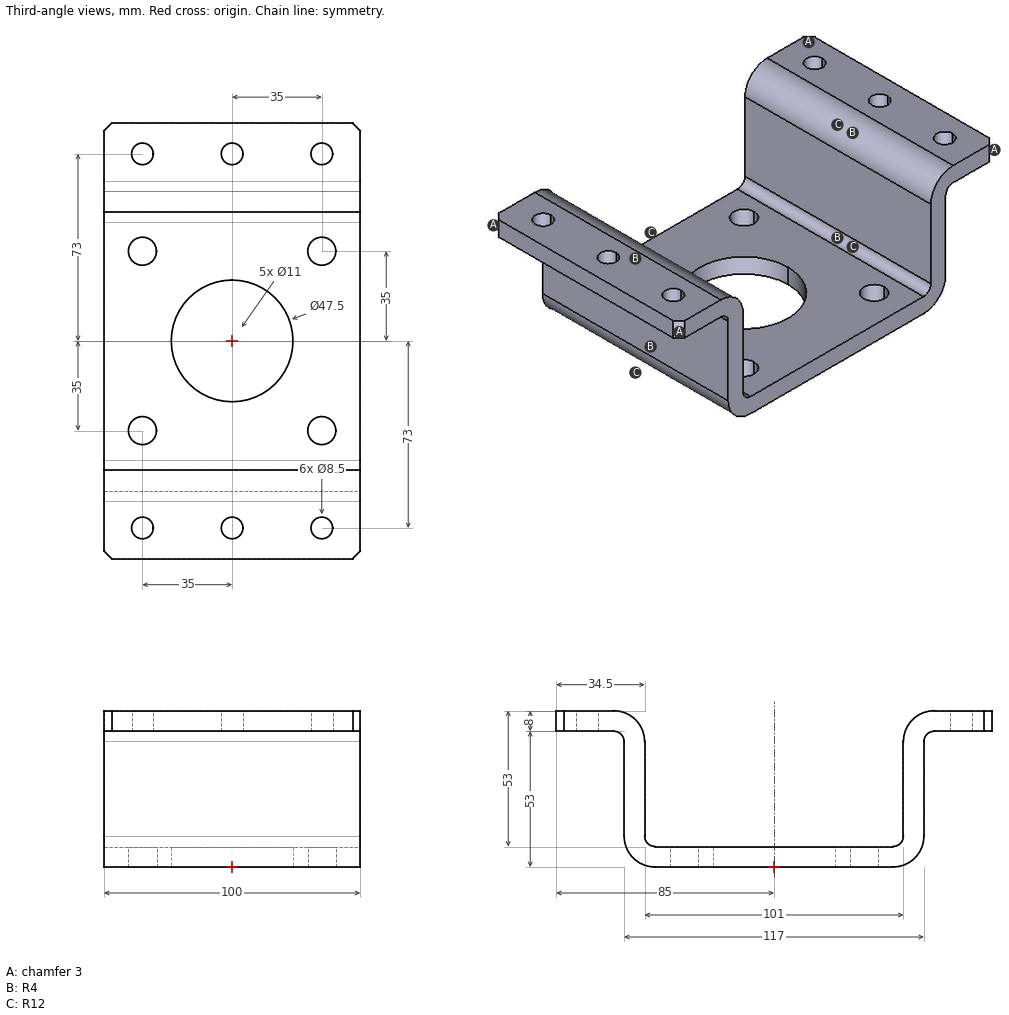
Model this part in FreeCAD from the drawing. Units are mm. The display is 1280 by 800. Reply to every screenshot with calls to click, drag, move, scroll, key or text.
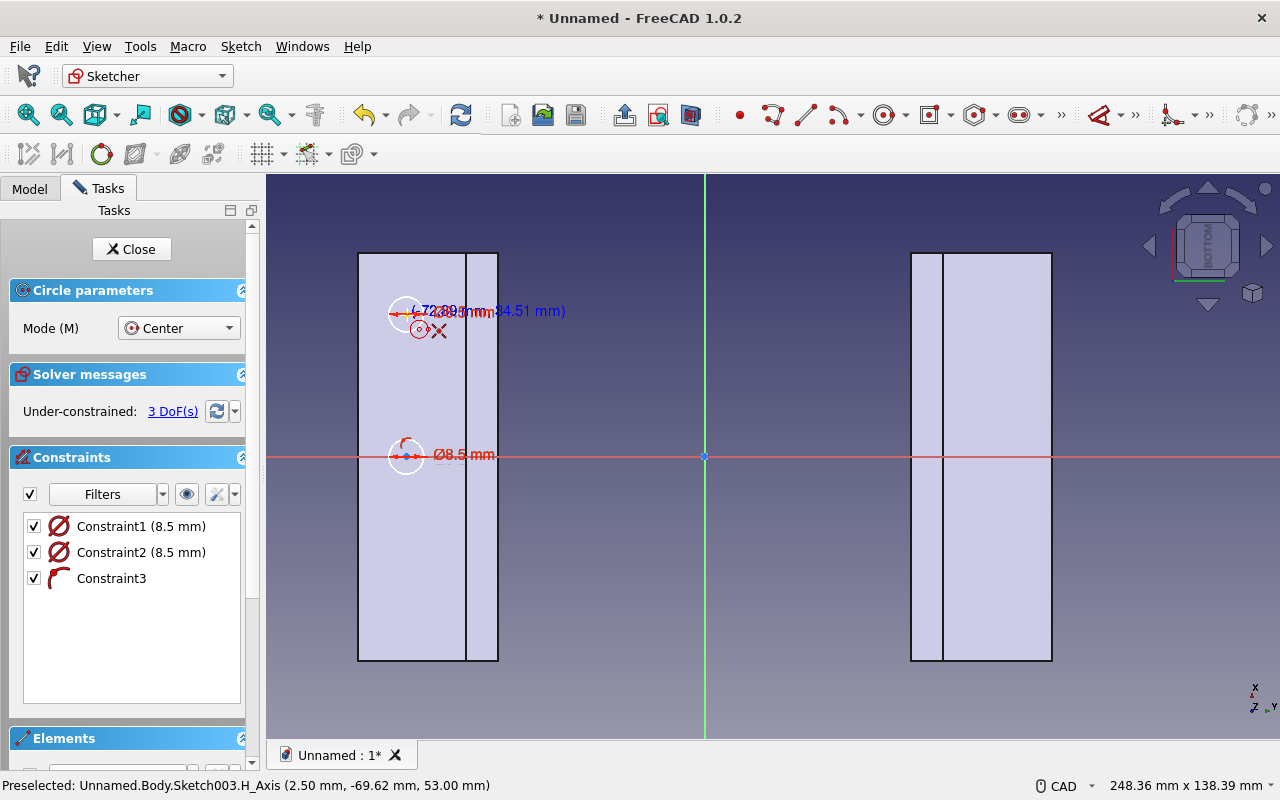
scroll(407, 600, up, 2)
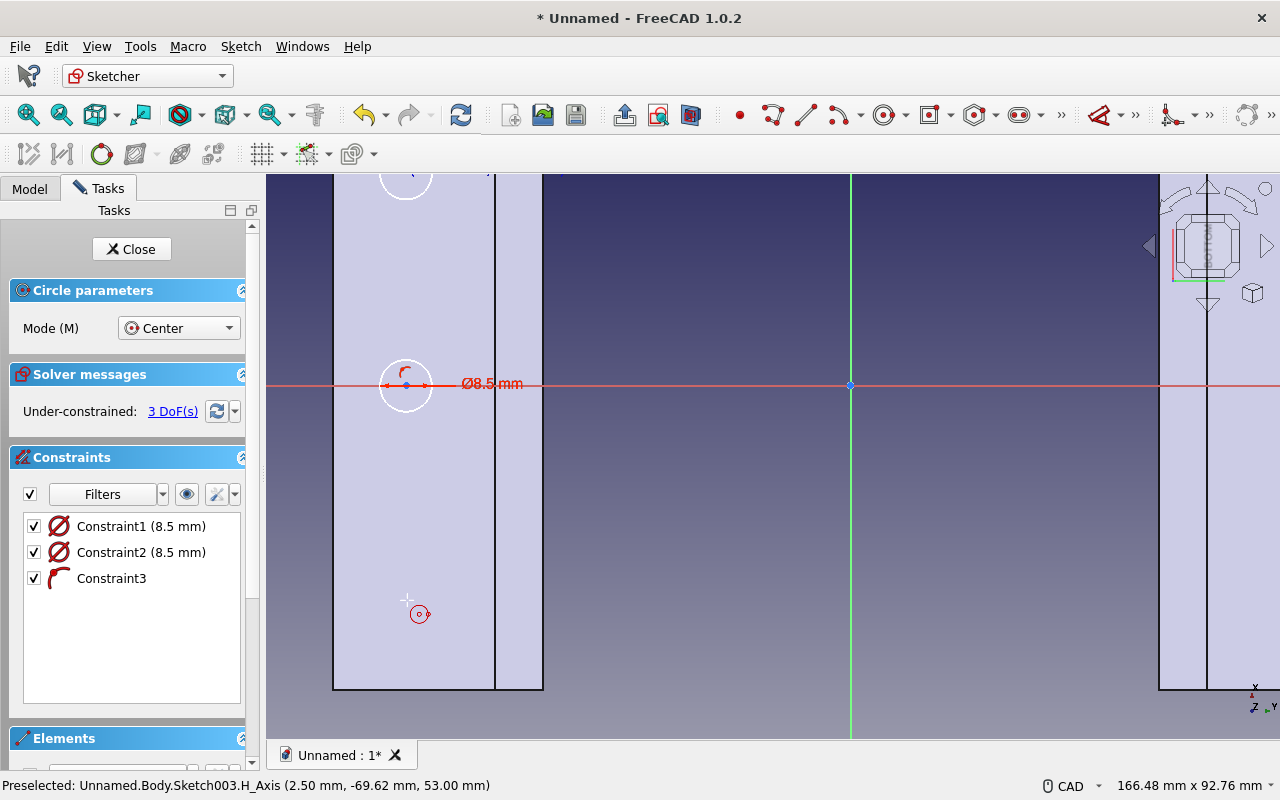
click(406, 599)
move(425, 581)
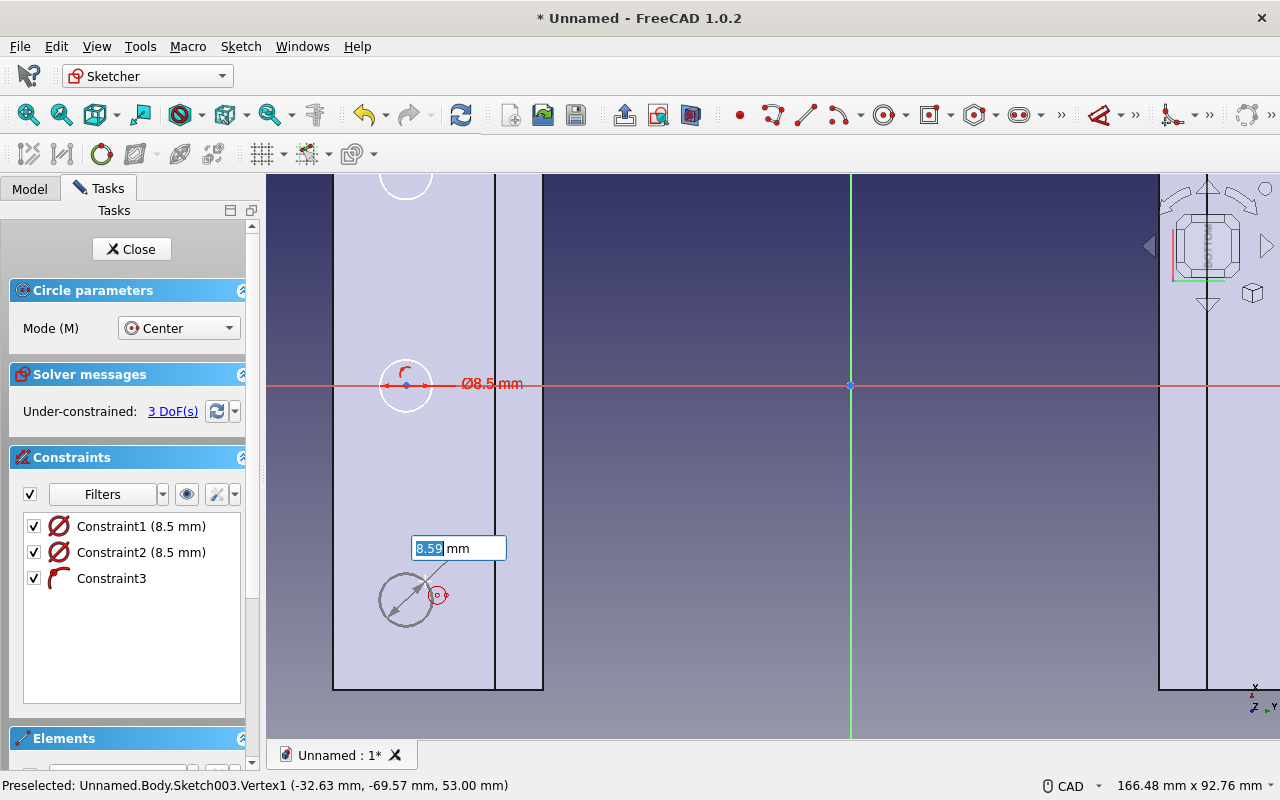
text(8.5)
key(Return)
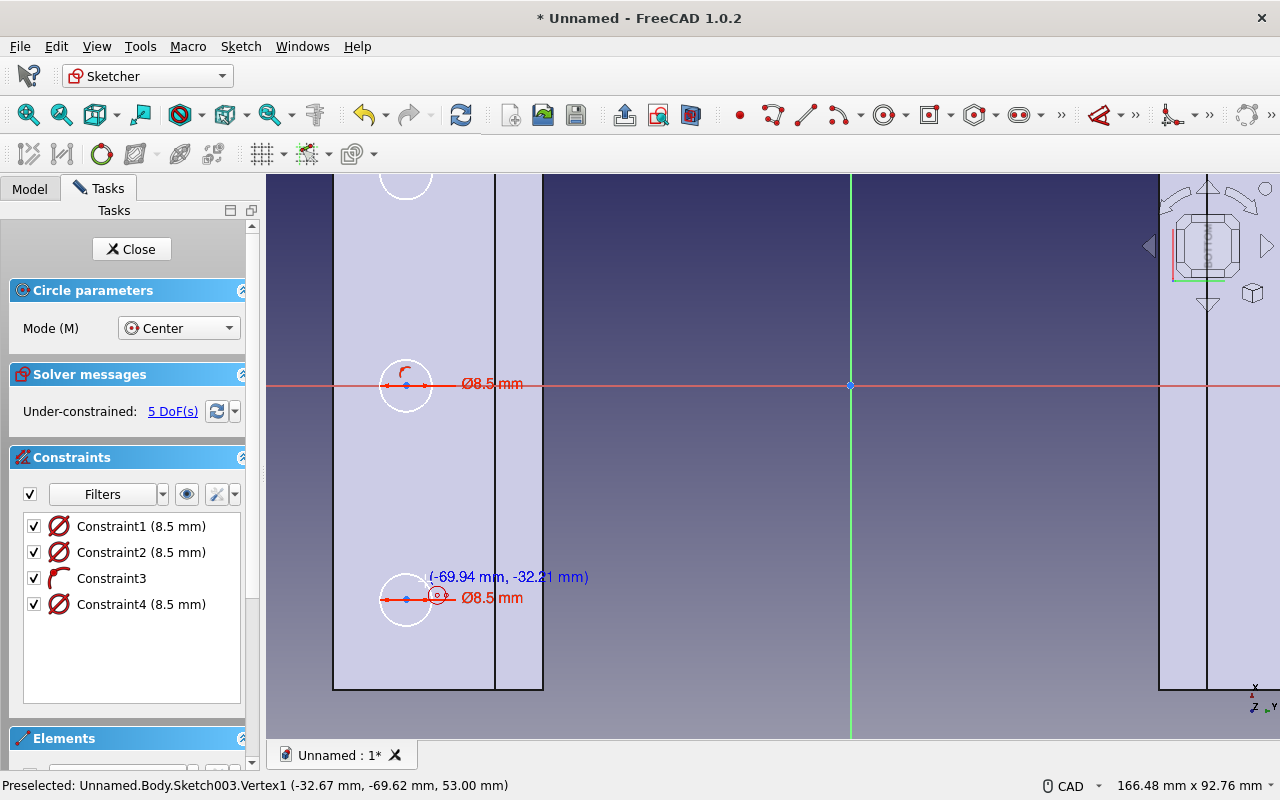
scroll(407, 600, down, 2)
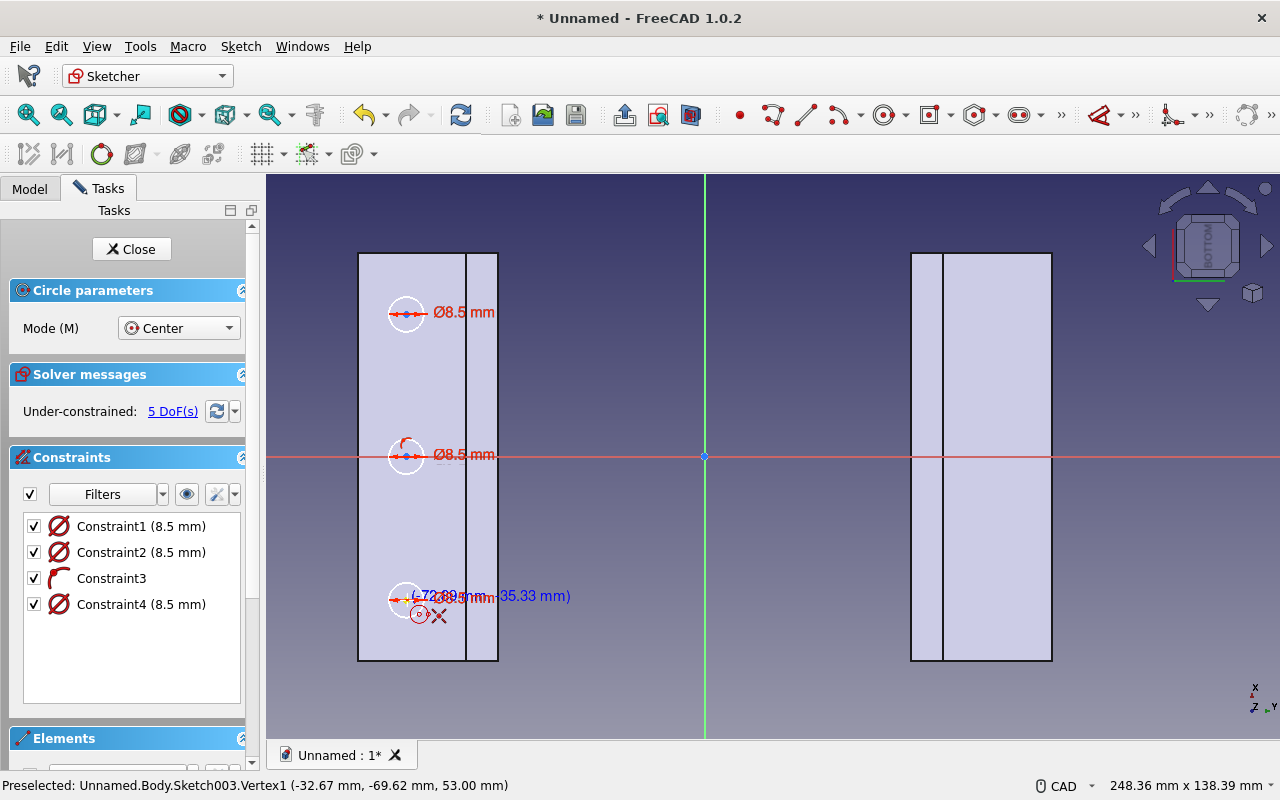
scroll(1003, 600, up, 2)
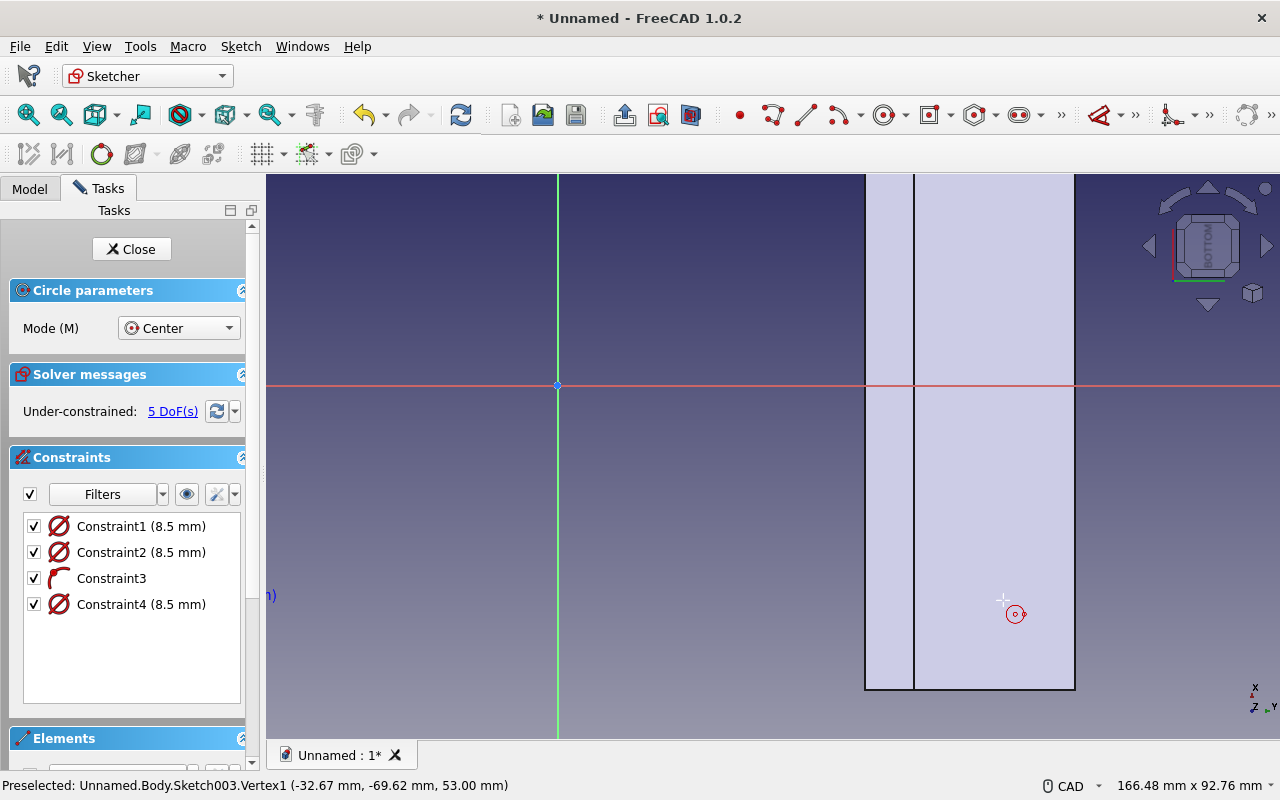
click(1002, 599)
move(1020, 581)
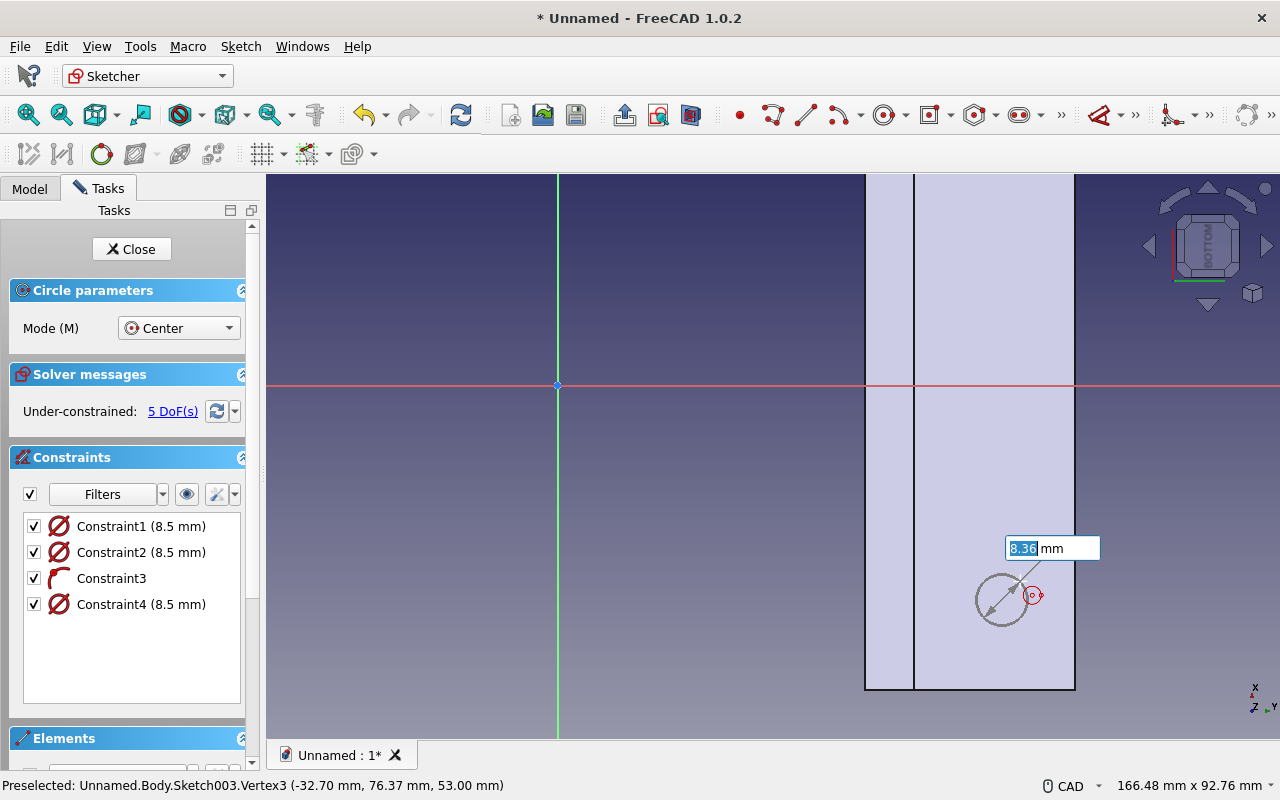
text(8.5)
key(Return)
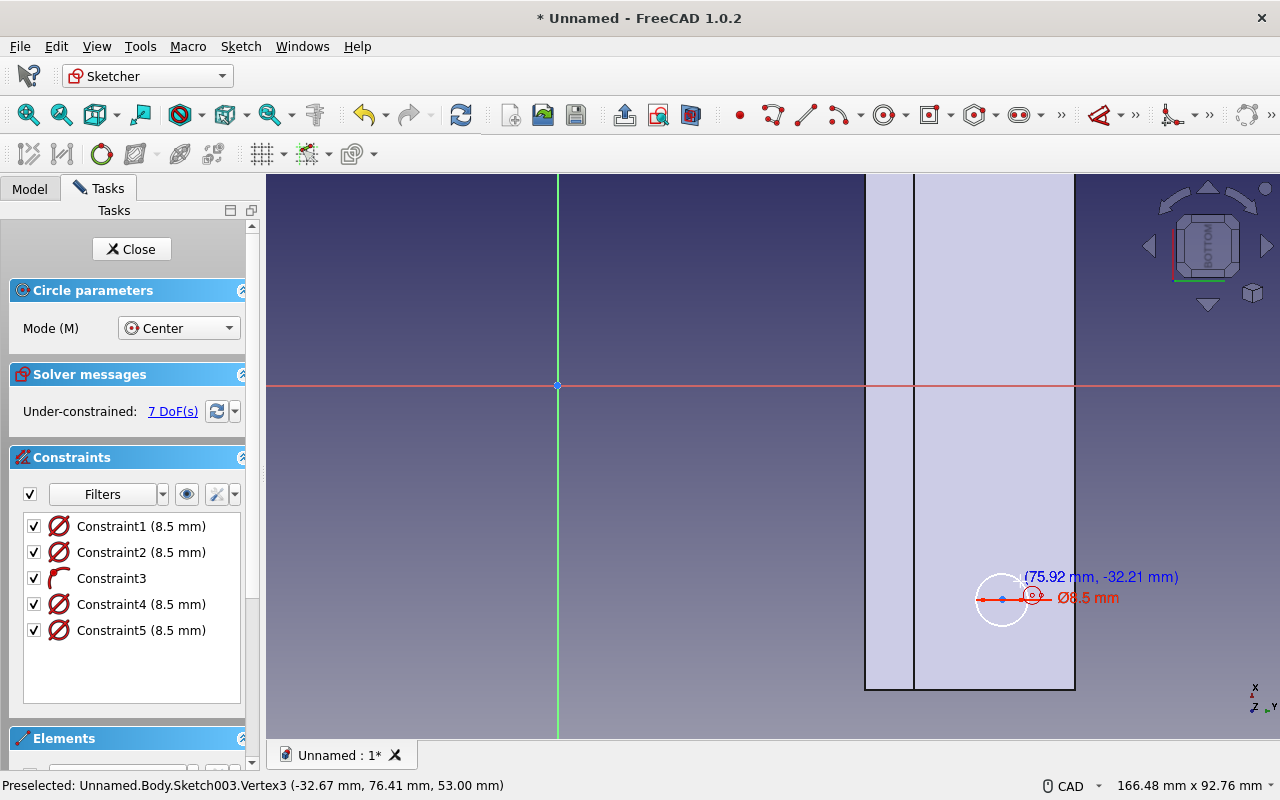
click(1002, 386)
move(1020, 367)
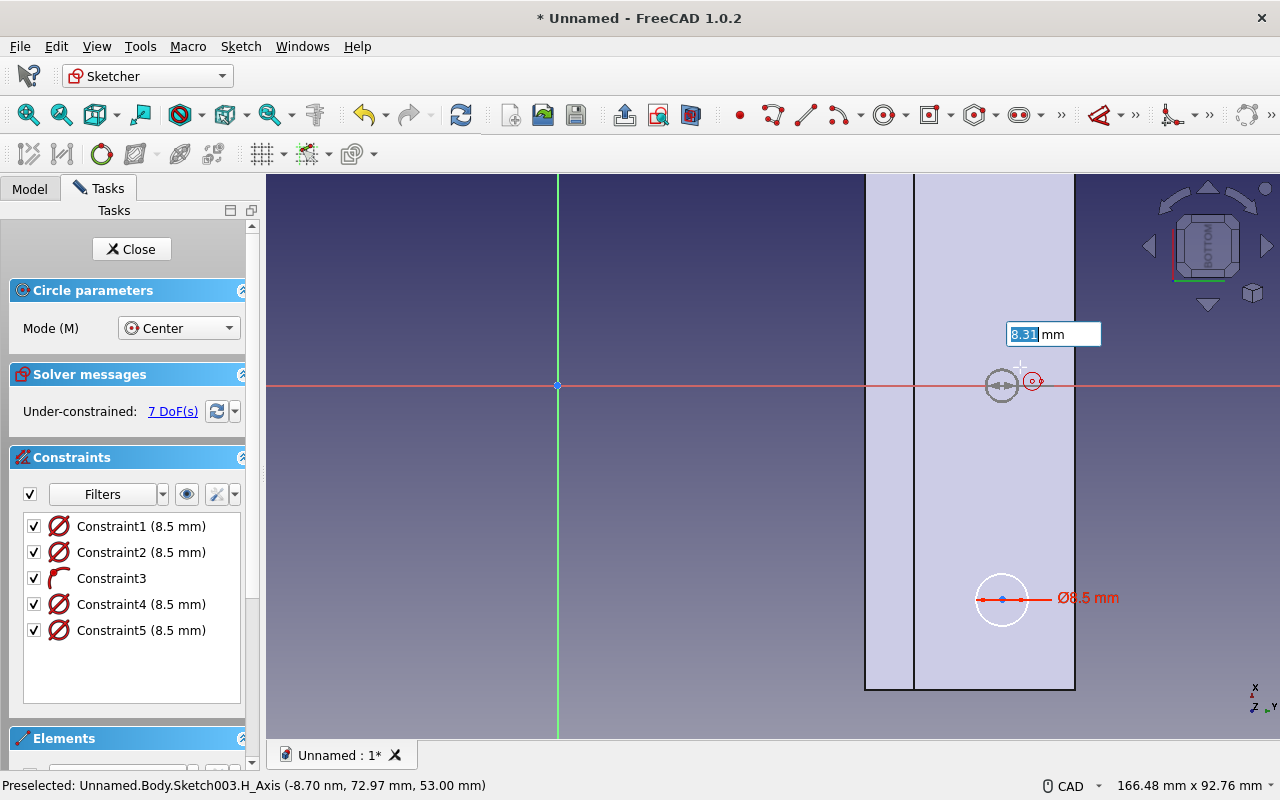
text(8.5)
key(Return)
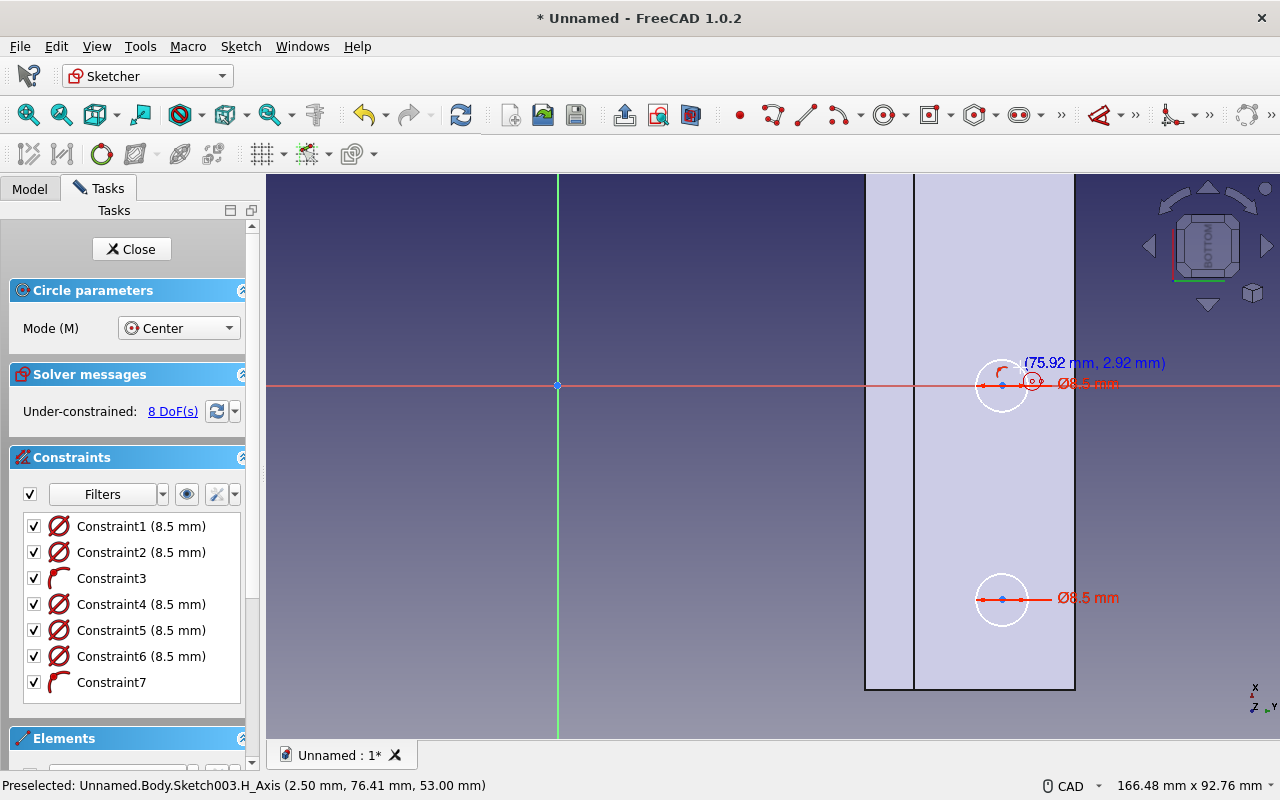
scroll(1003, 600, down, 2)